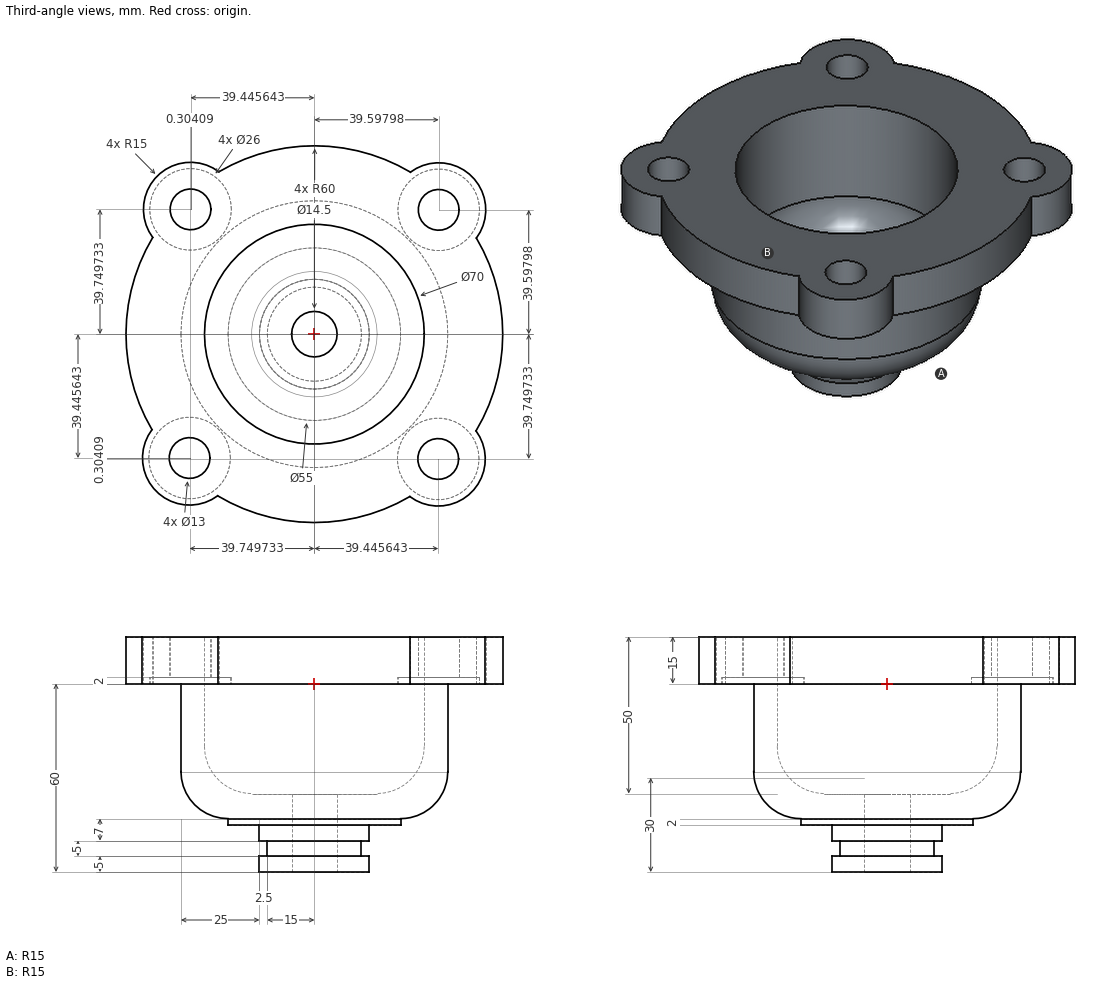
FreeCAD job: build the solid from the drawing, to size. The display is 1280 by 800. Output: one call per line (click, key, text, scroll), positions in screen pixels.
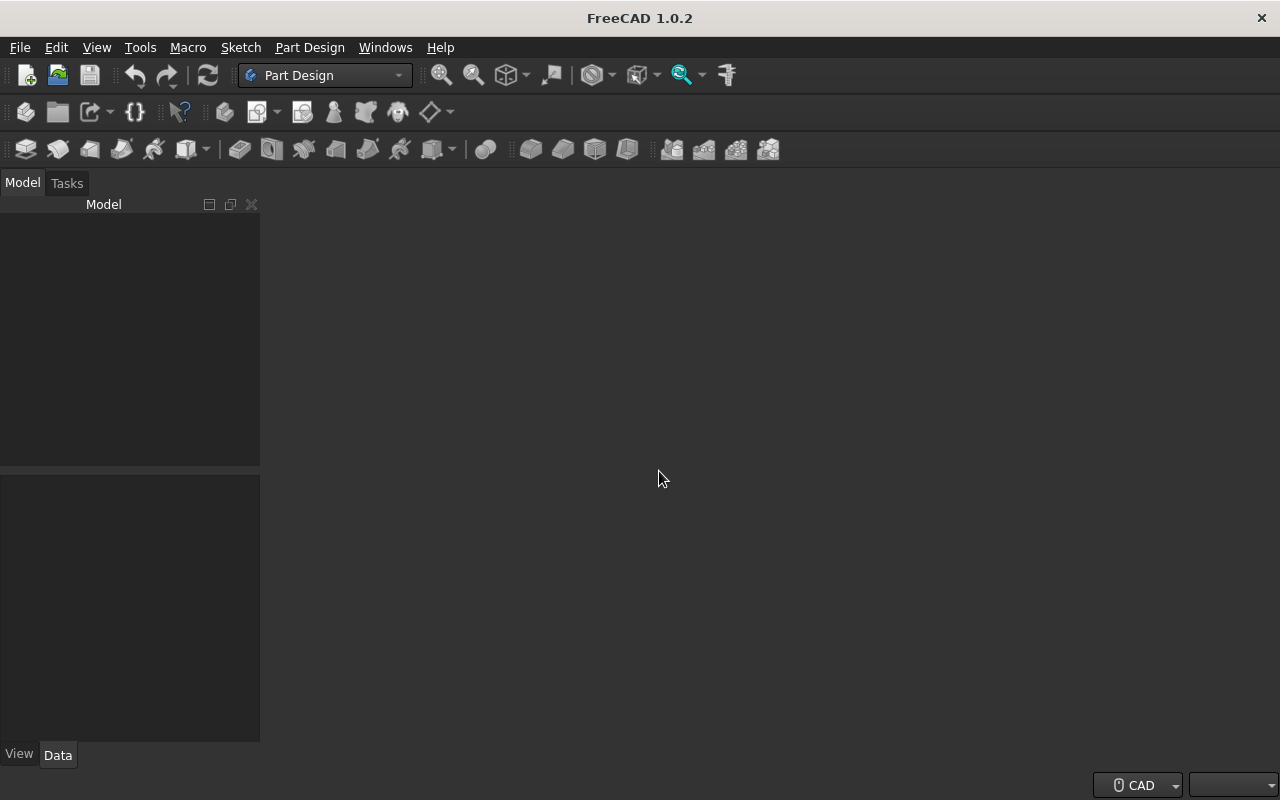
click(26, 76)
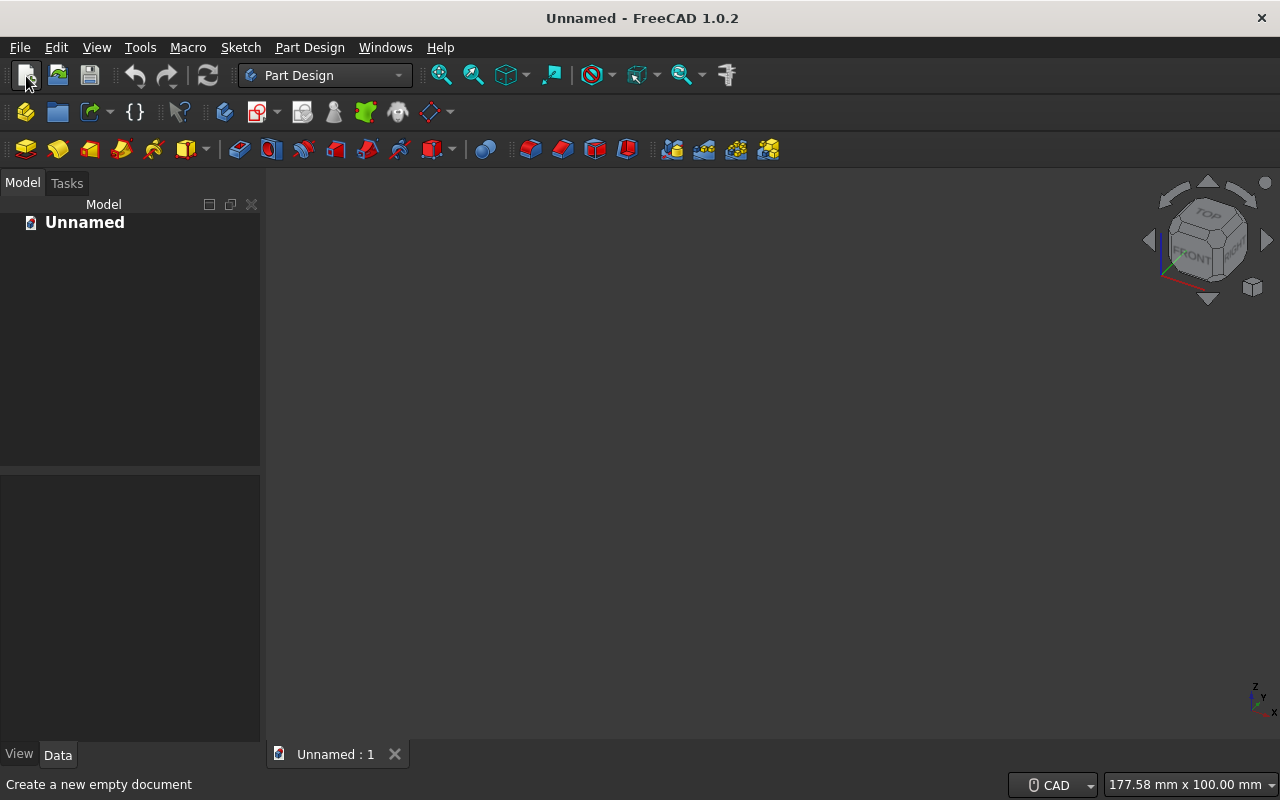
click(258, 112)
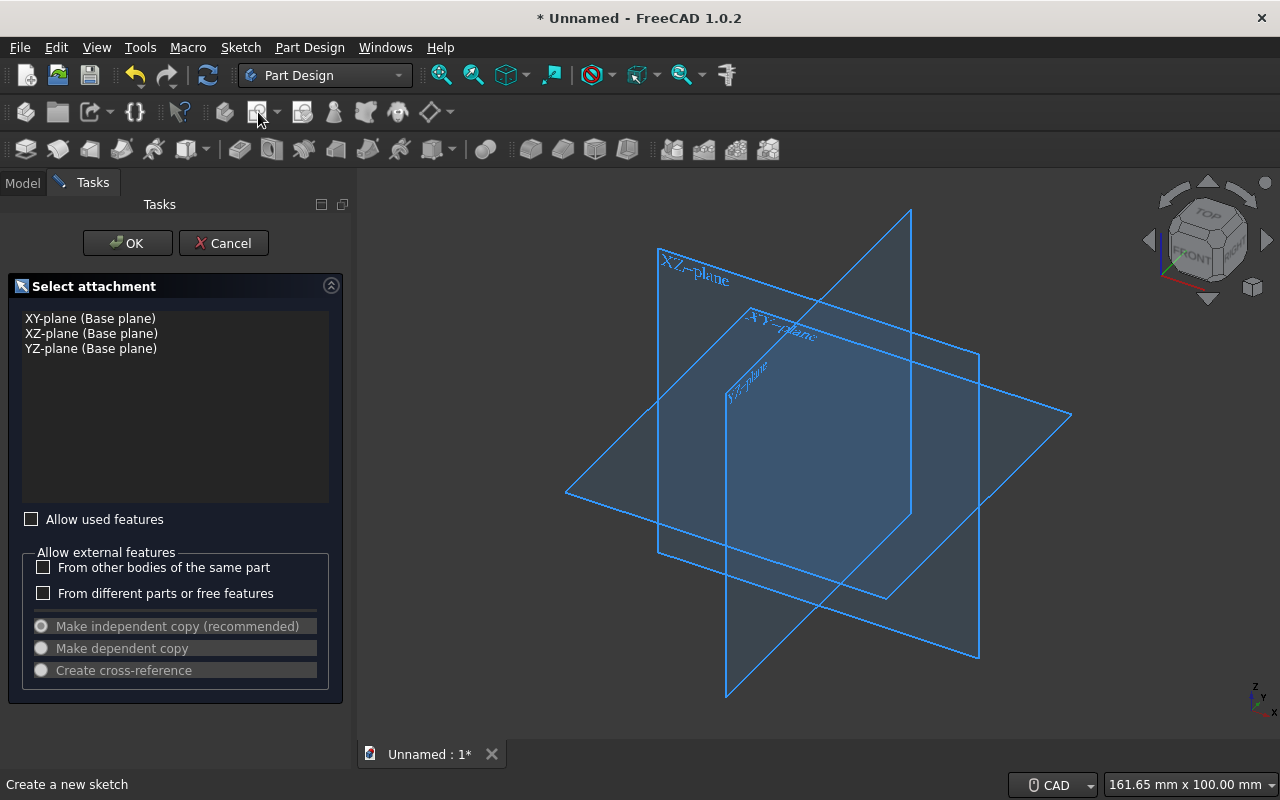
click(82, 318)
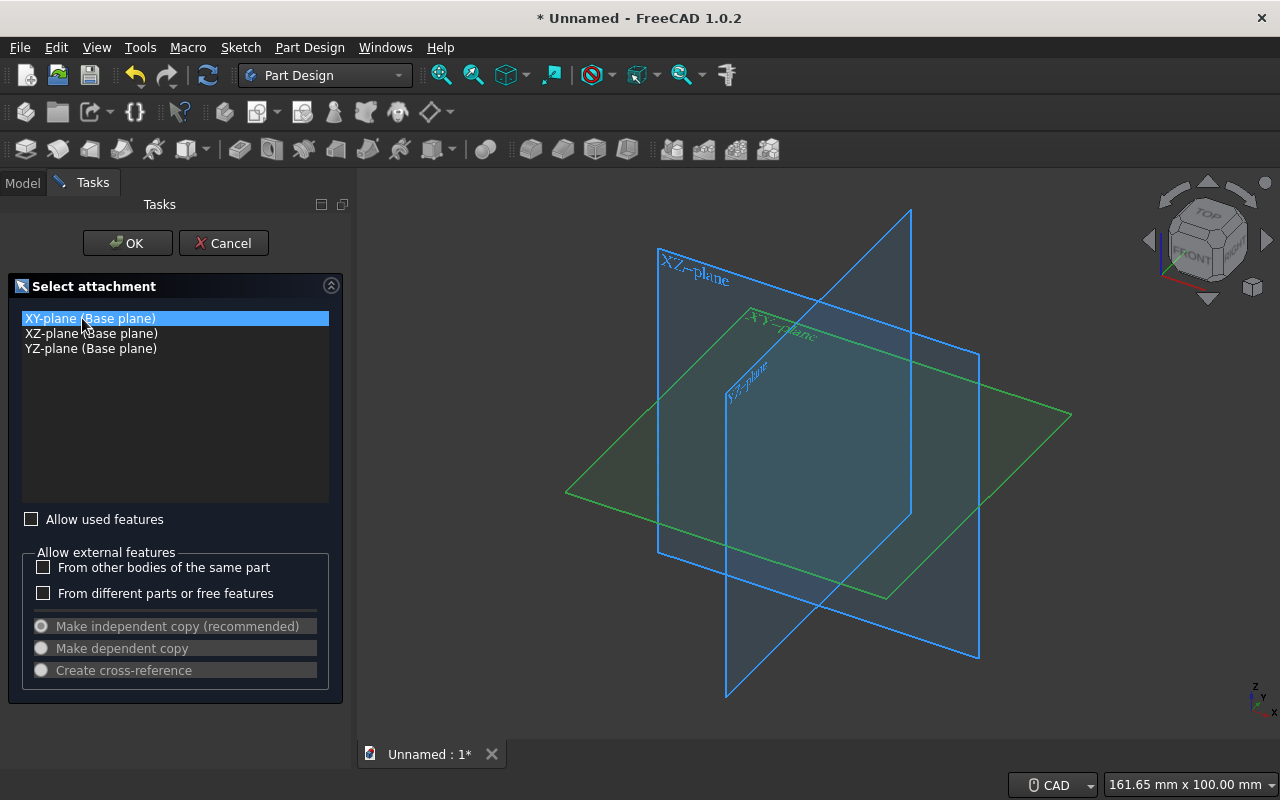
click(128, 243)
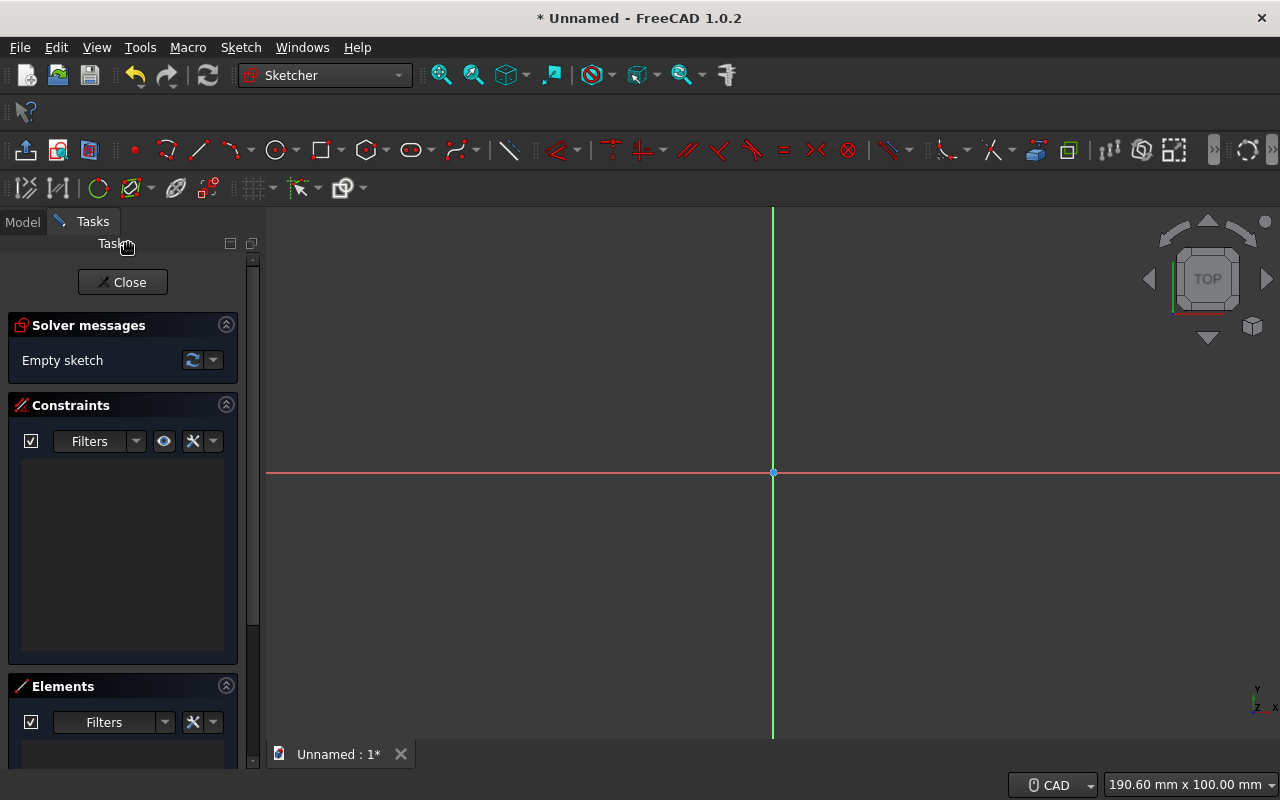
scroll(621, 473, down, 3)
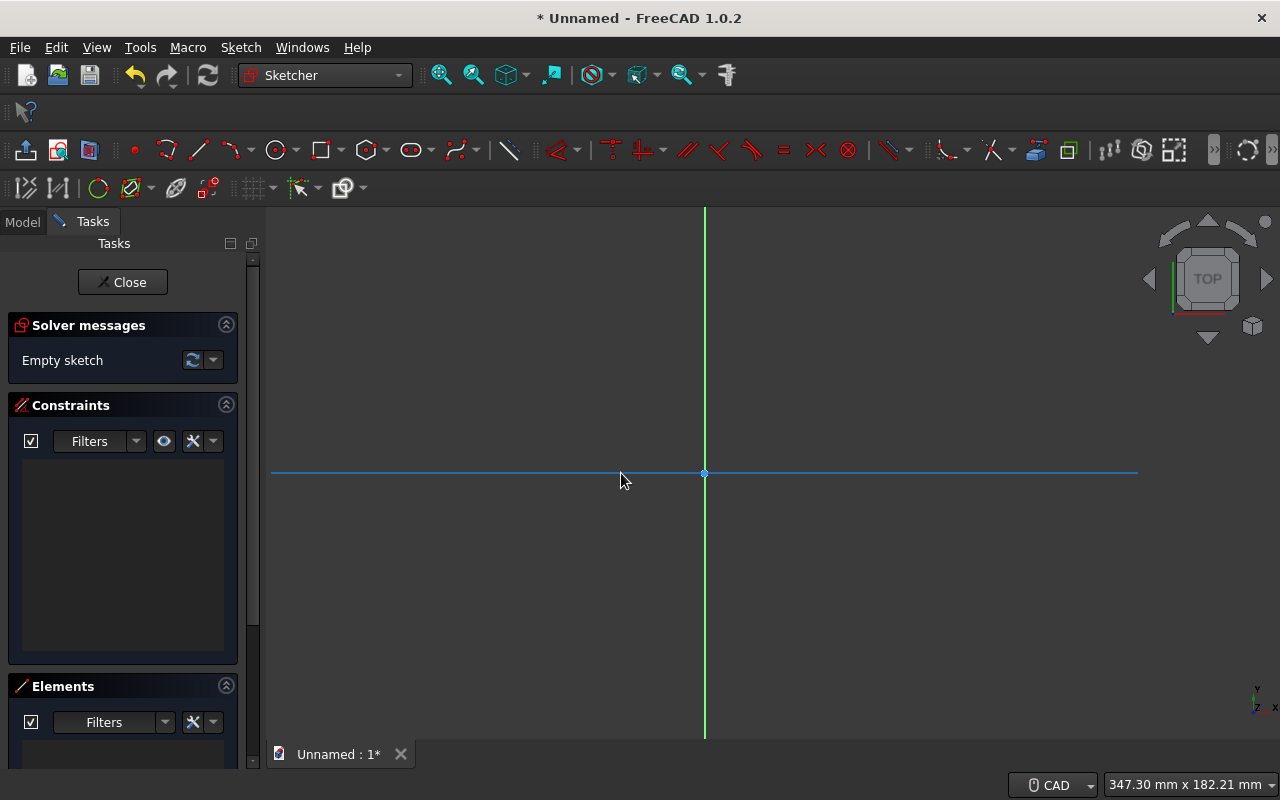
click(232, 150)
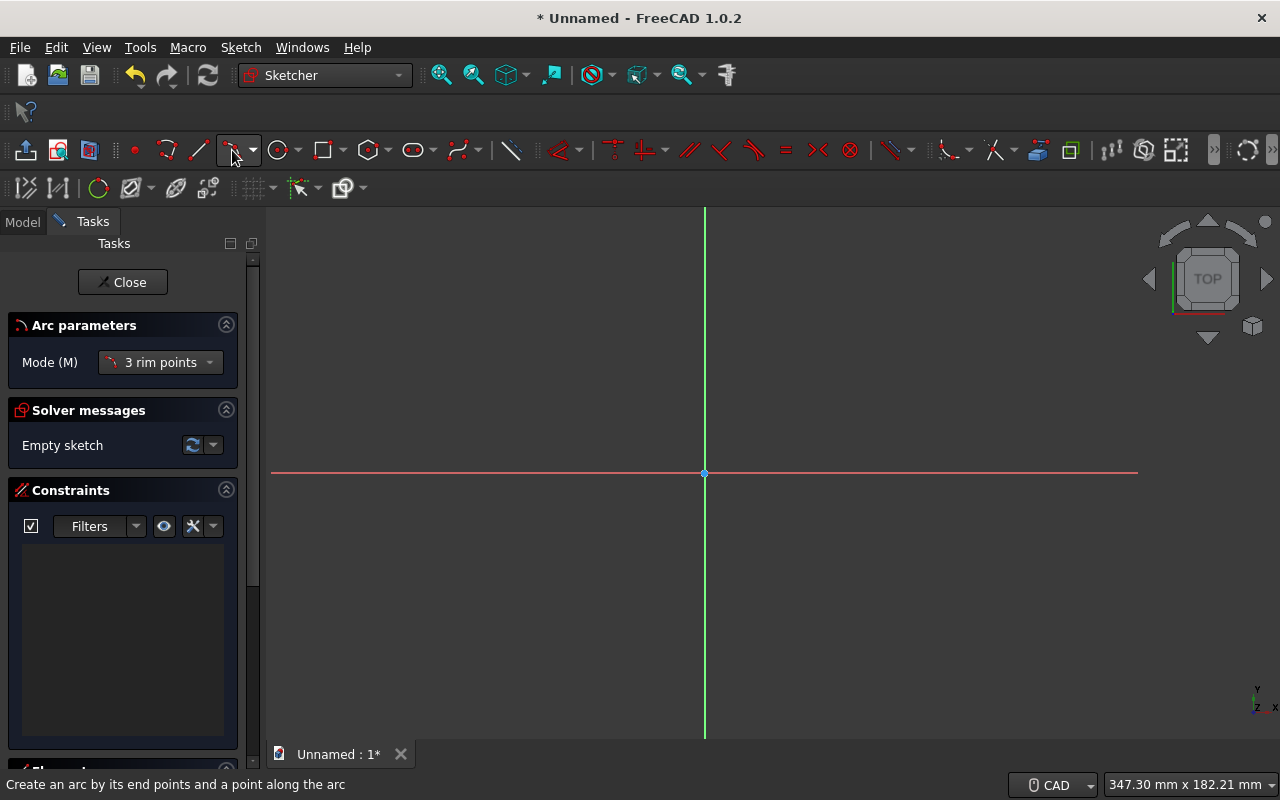
click(616, 322)
click(554, 383)
click(559, 326)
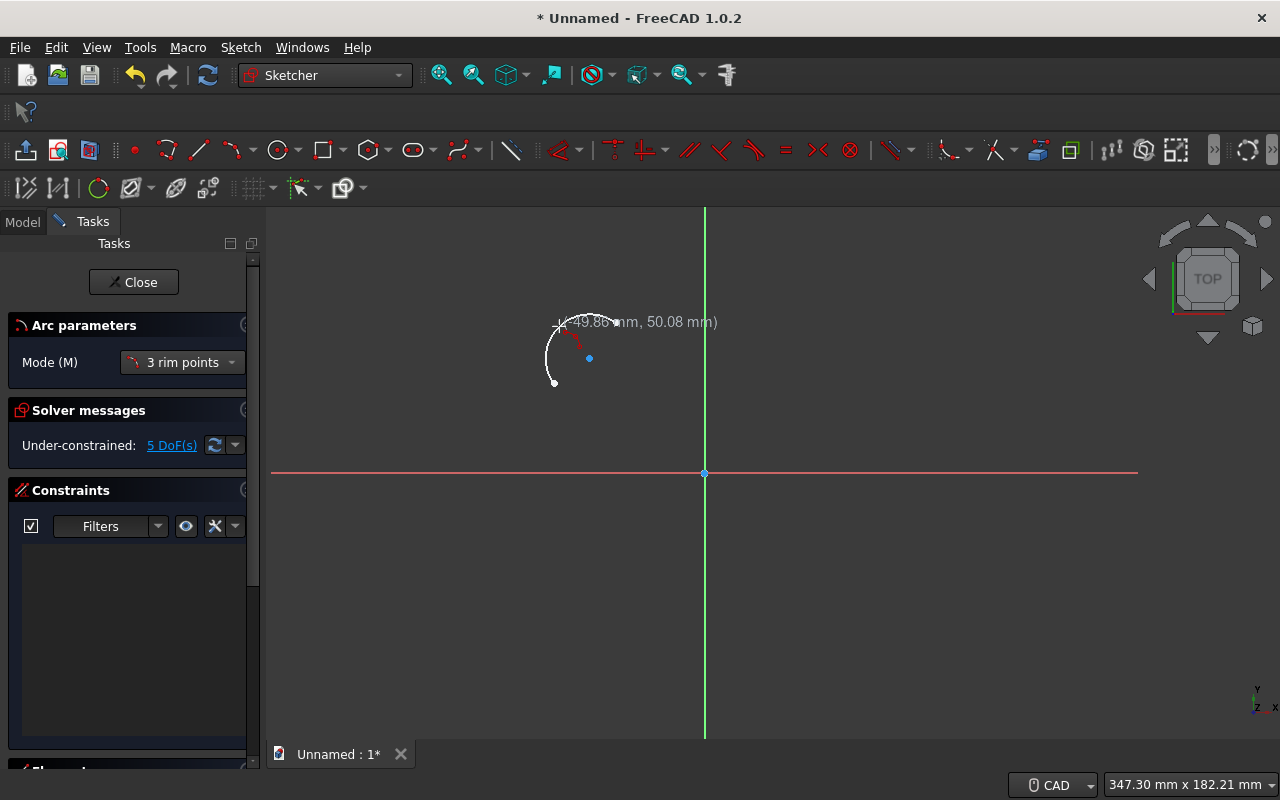
click(554, 384)
click(554, 562)
click(530, 454)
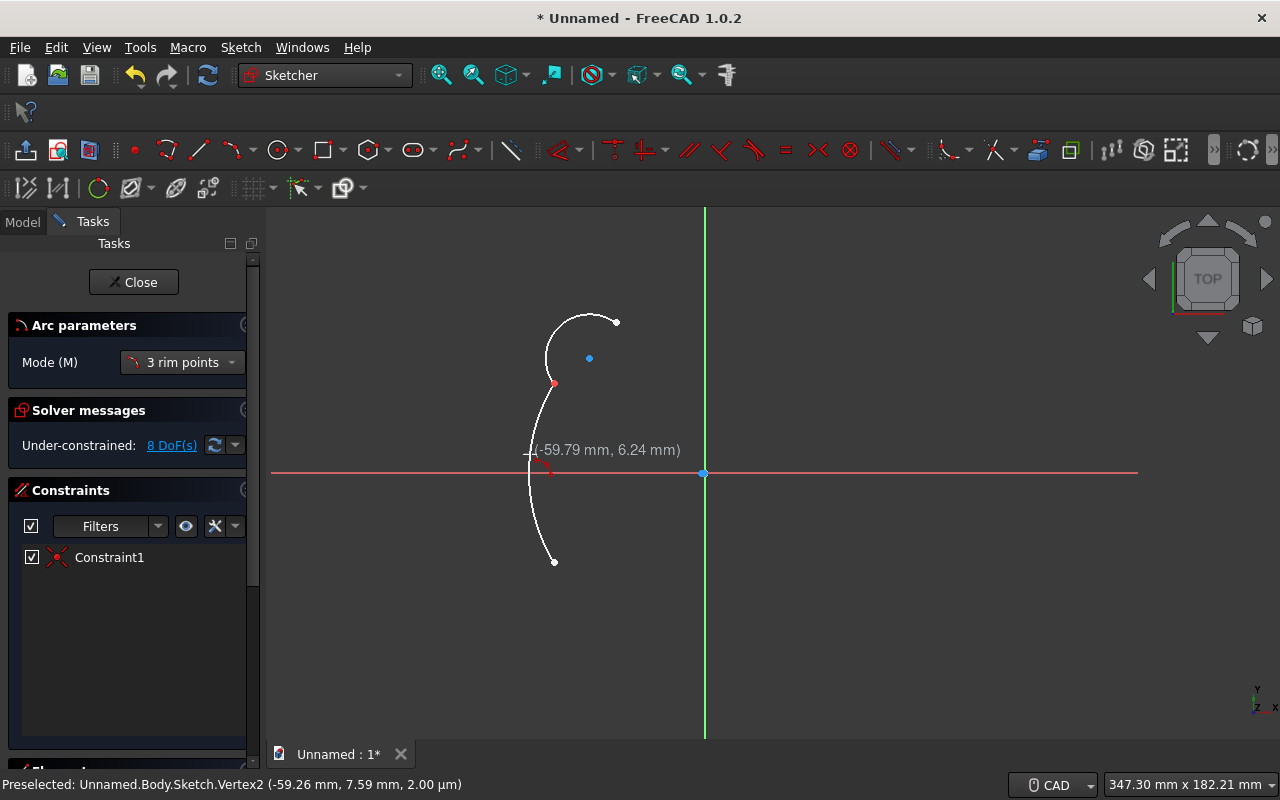
click(554, 563)
click(615, 624)
click(557, 619)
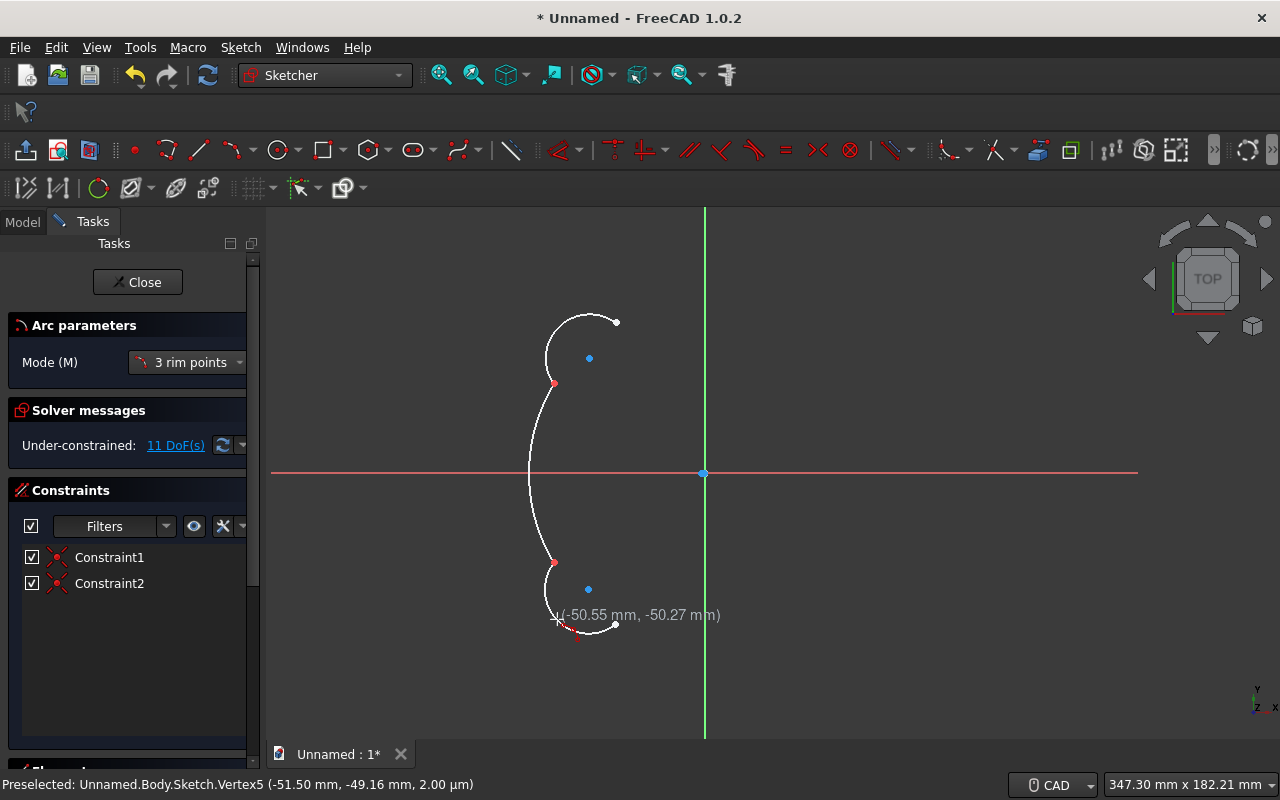
click(615, 625)
click(793, 624)
click(685, 647)